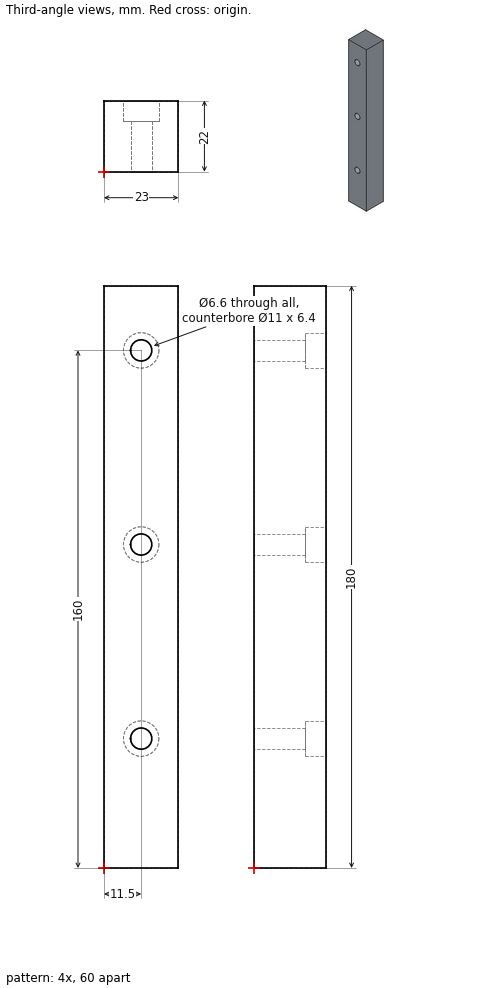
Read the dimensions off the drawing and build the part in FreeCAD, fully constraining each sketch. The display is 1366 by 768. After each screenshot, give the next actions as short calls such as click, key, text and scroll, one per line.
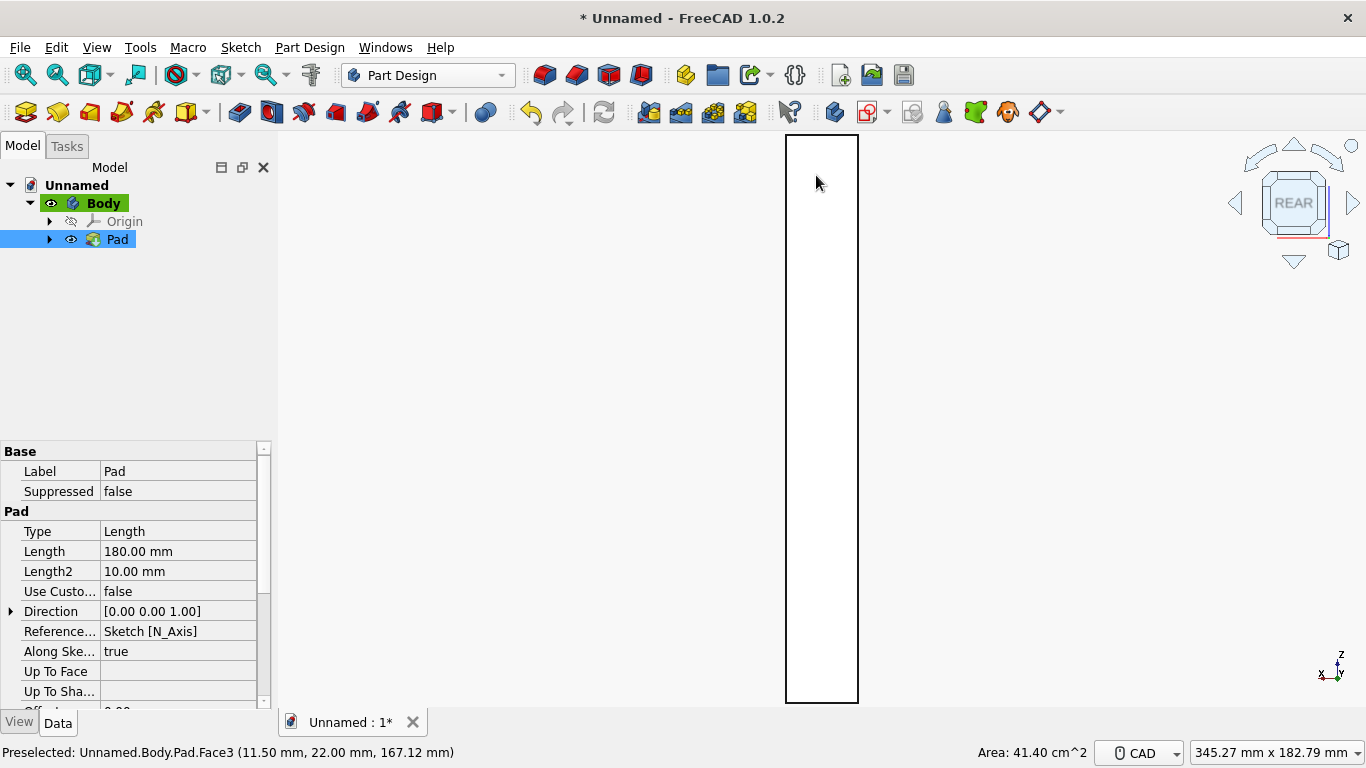
click(868, 112)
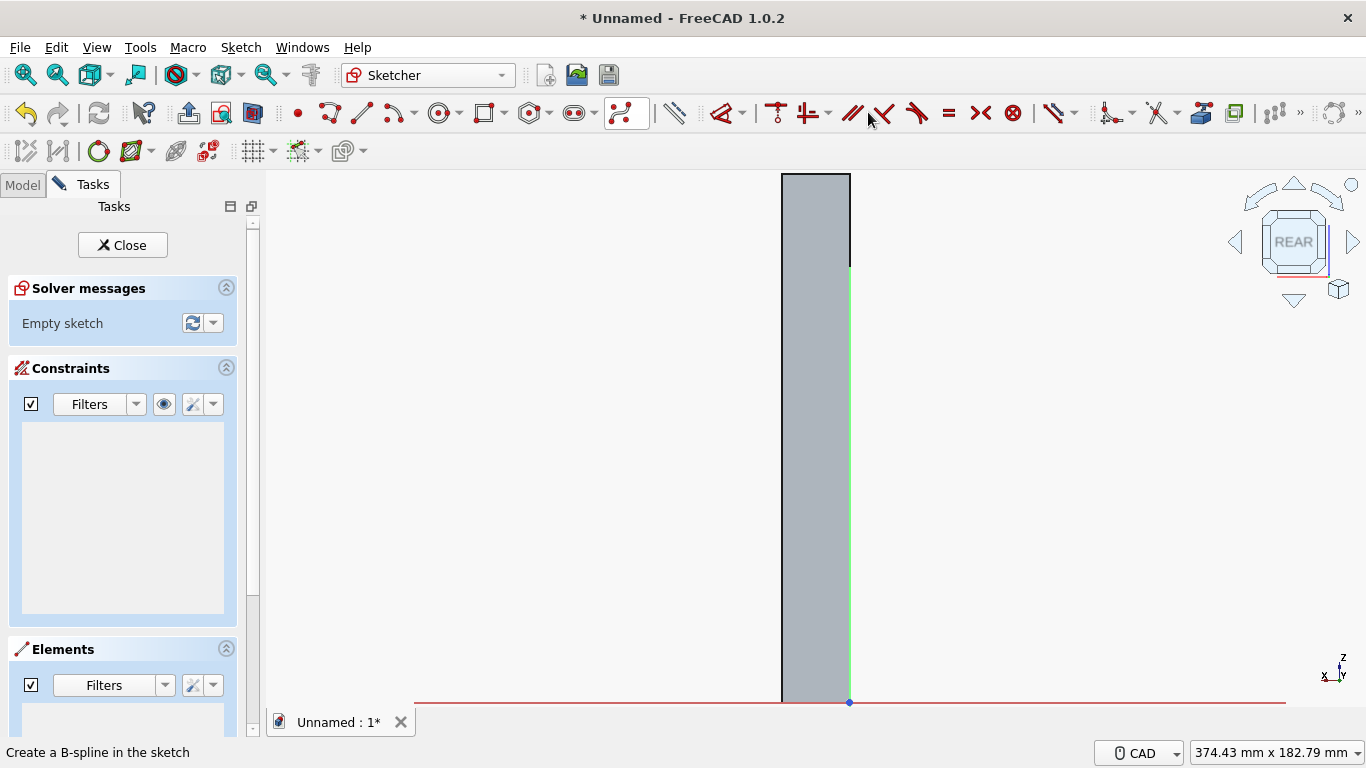
scroll(820, 220, up, 14)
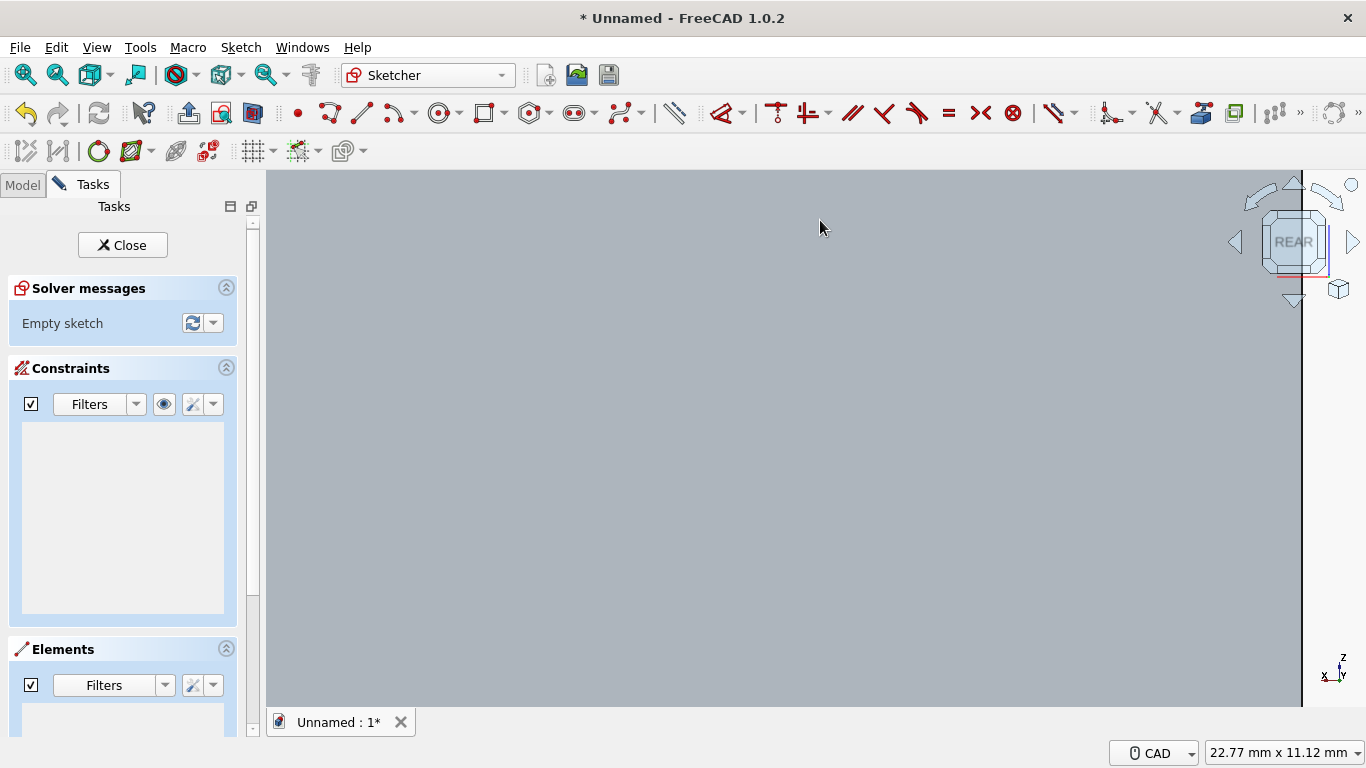
click(440, 114)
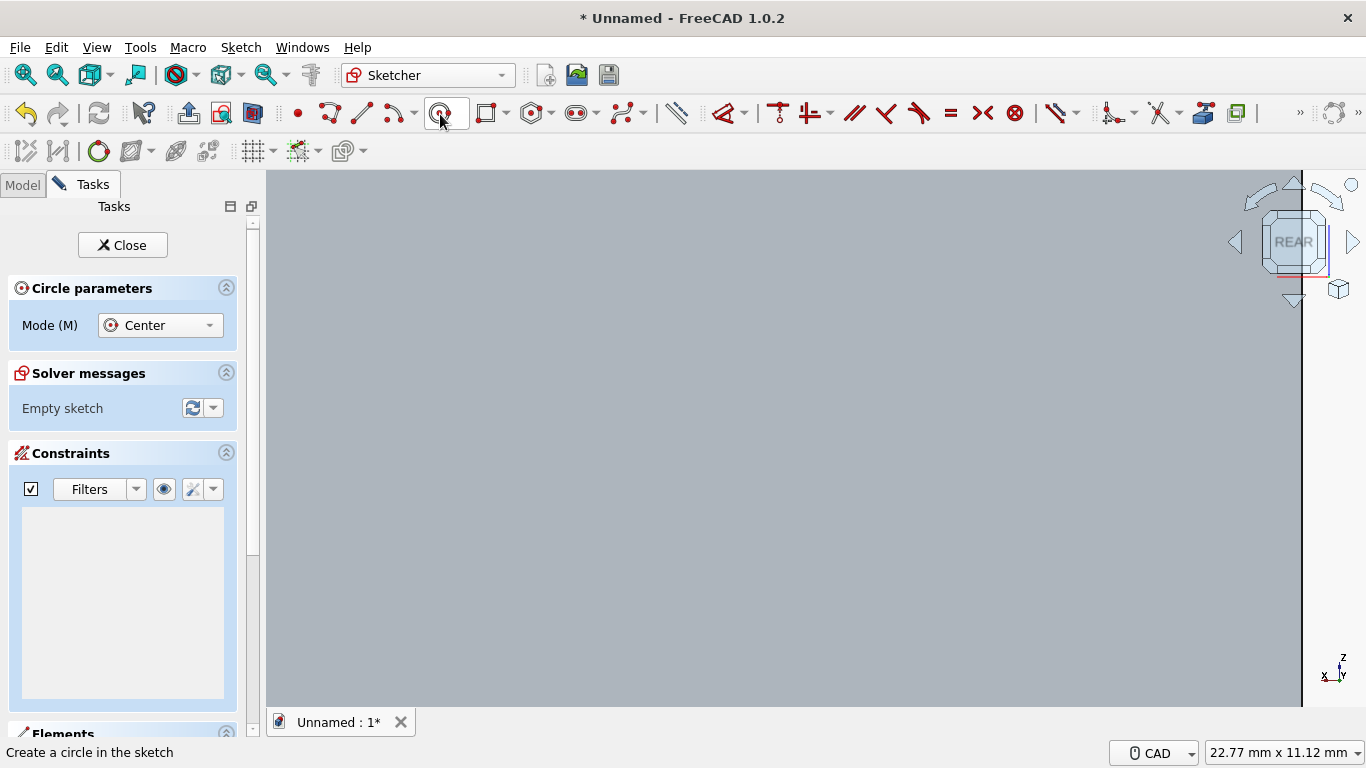
click(746, 430)
click(859, 317)
key(Escape)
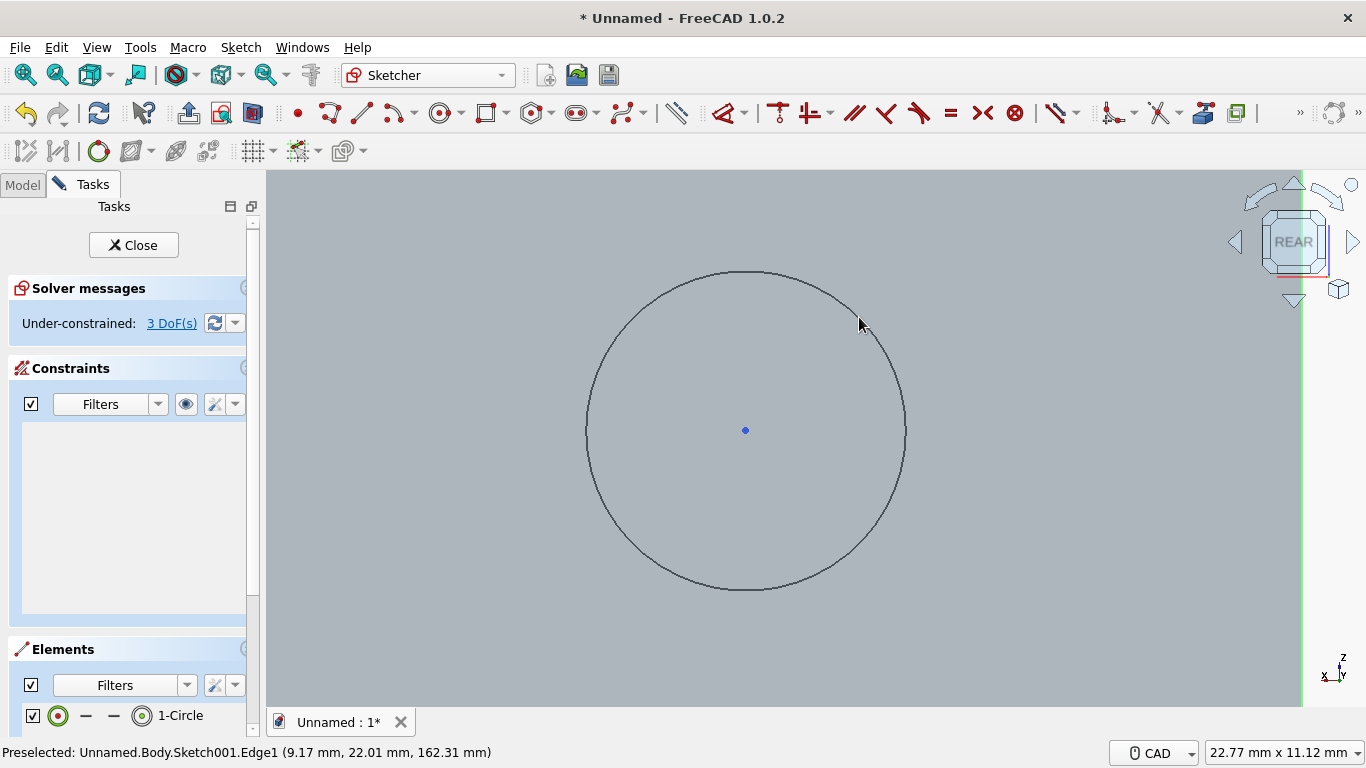
click(859, 318)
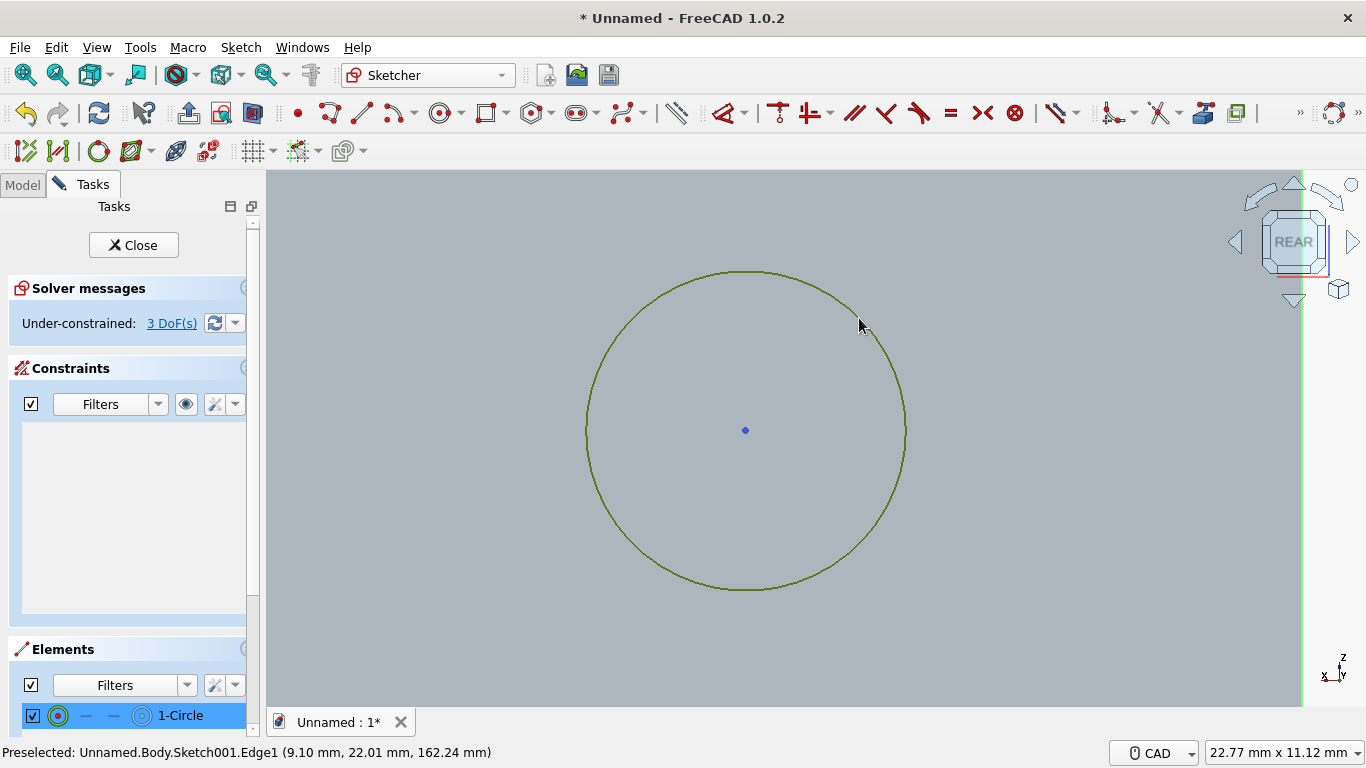
click(746, 114)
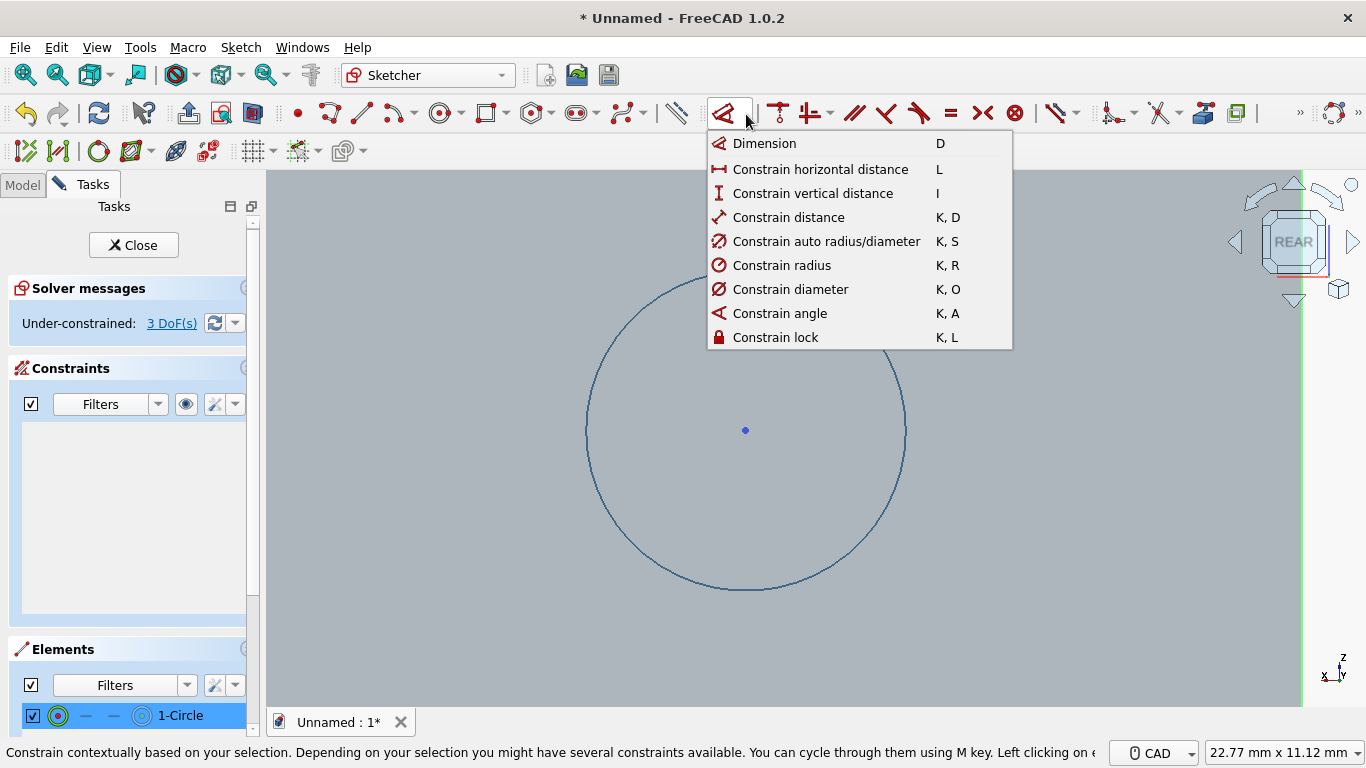
click(860, 289)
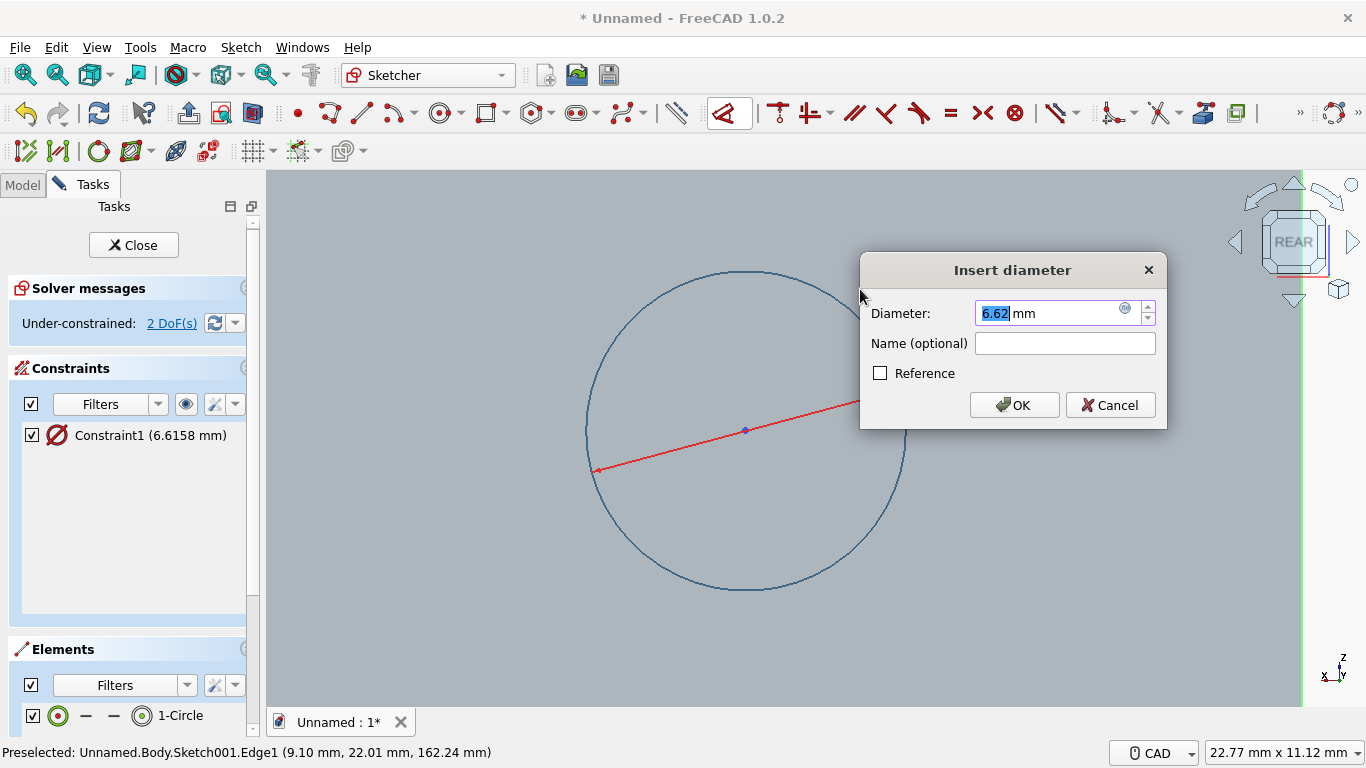
text(6.6)
key(Return)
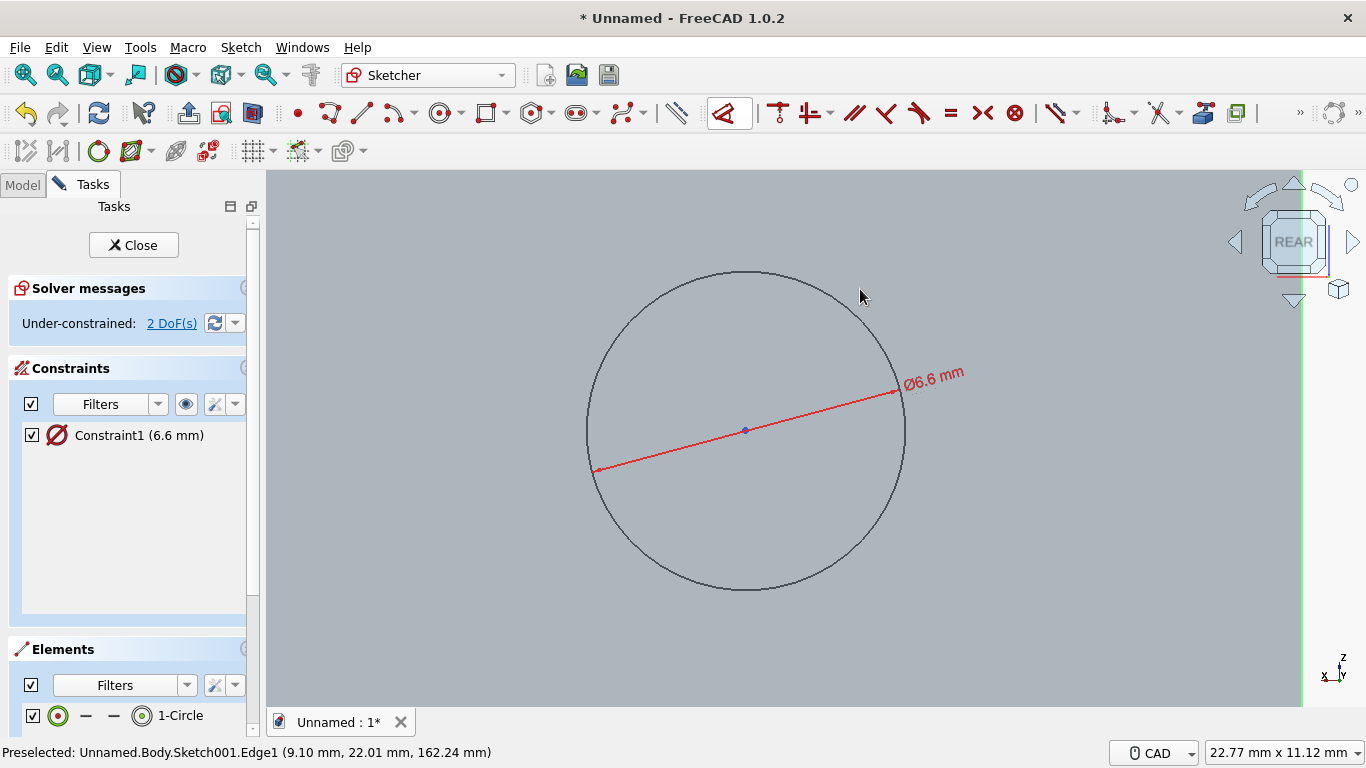
click(746, 431)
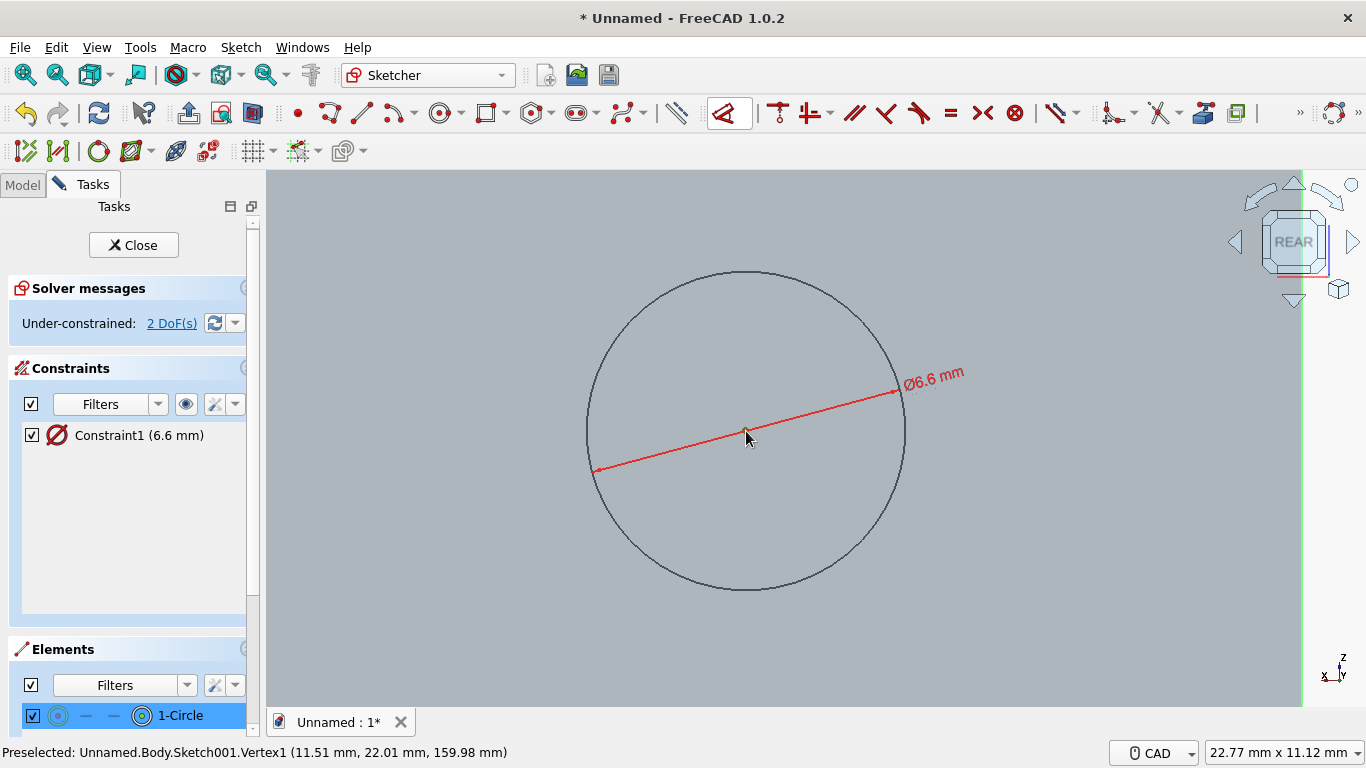
click(746, 114)